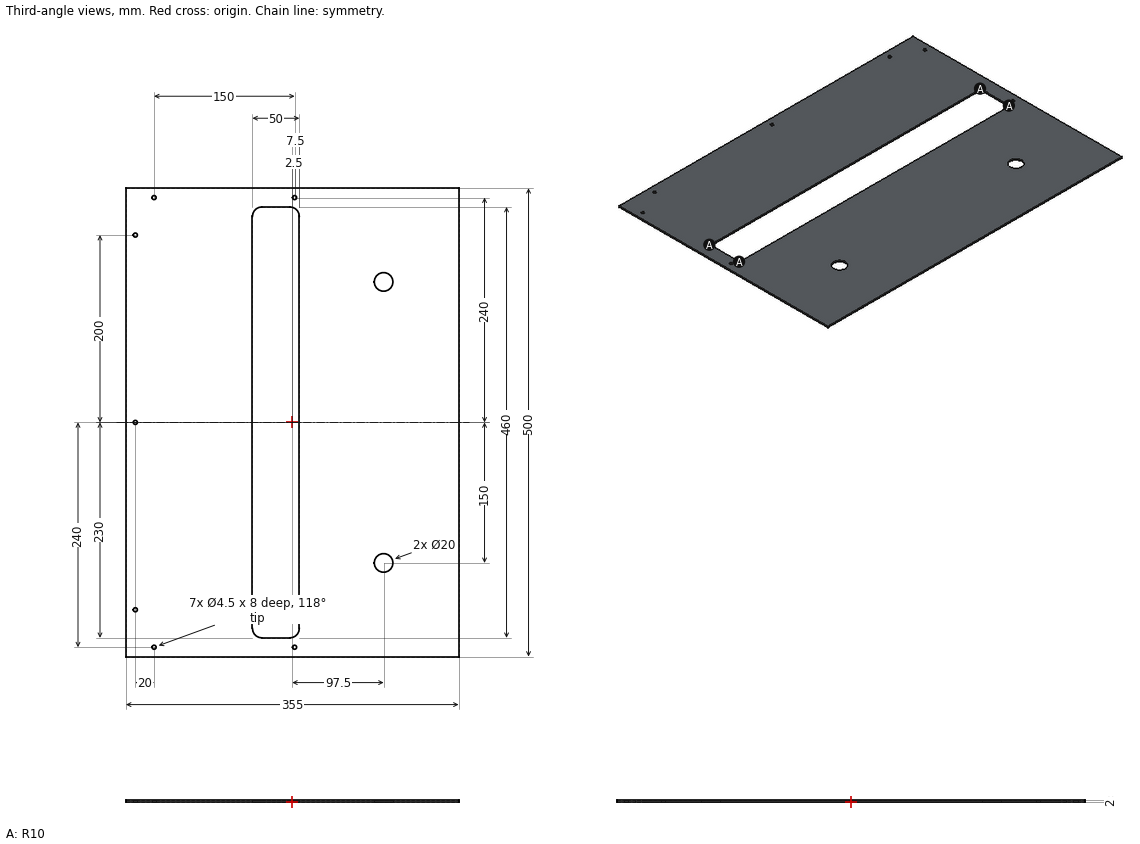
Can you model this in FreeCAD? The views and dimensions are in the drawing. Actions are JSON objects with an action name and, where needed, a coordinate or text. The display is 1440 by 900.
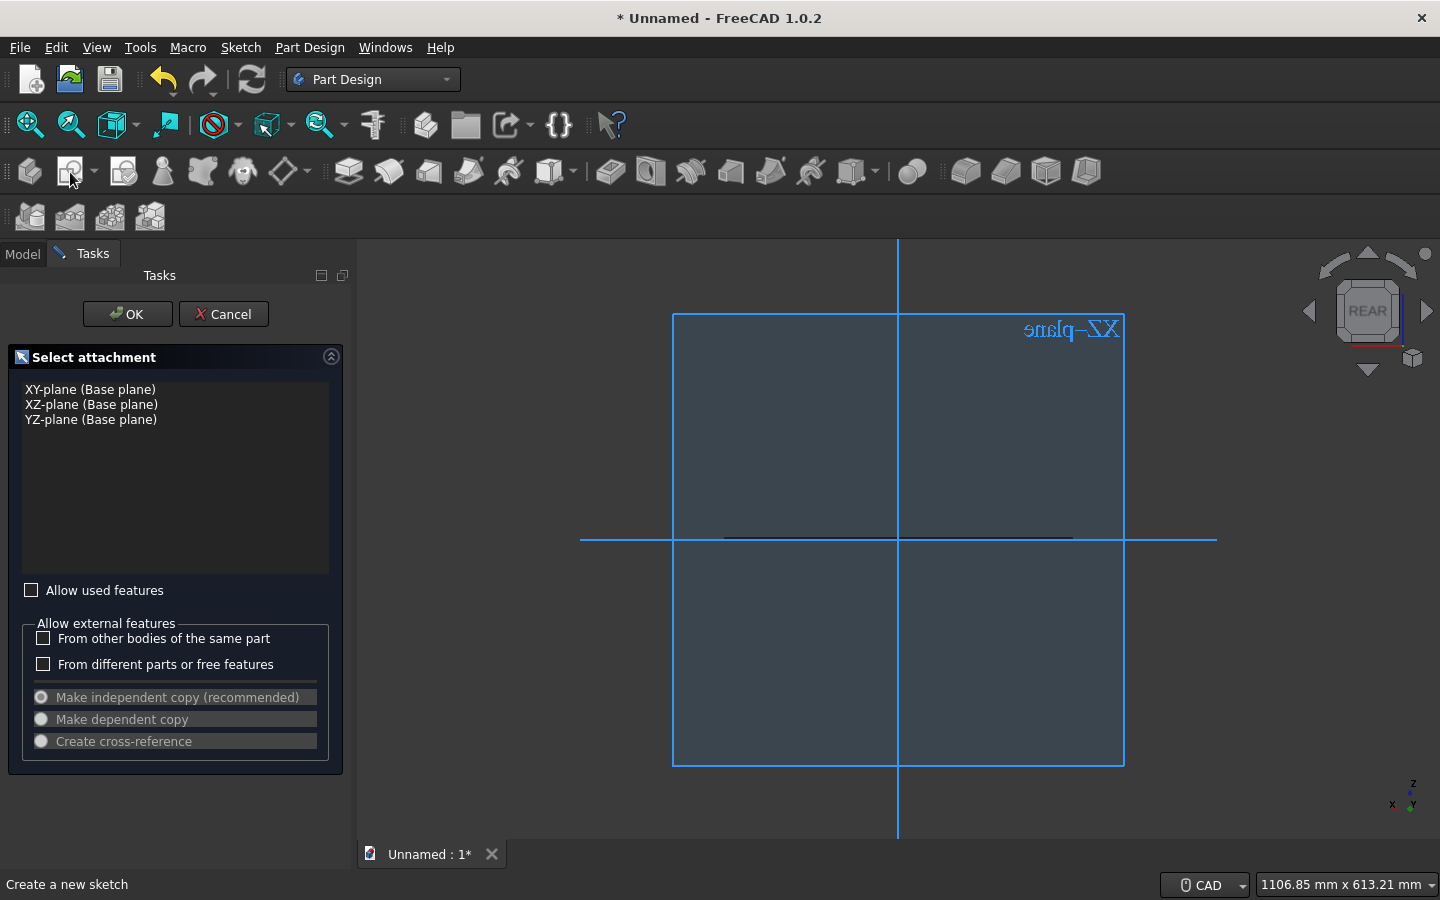
{"action": "left_click", "coordinate": [82, 390]}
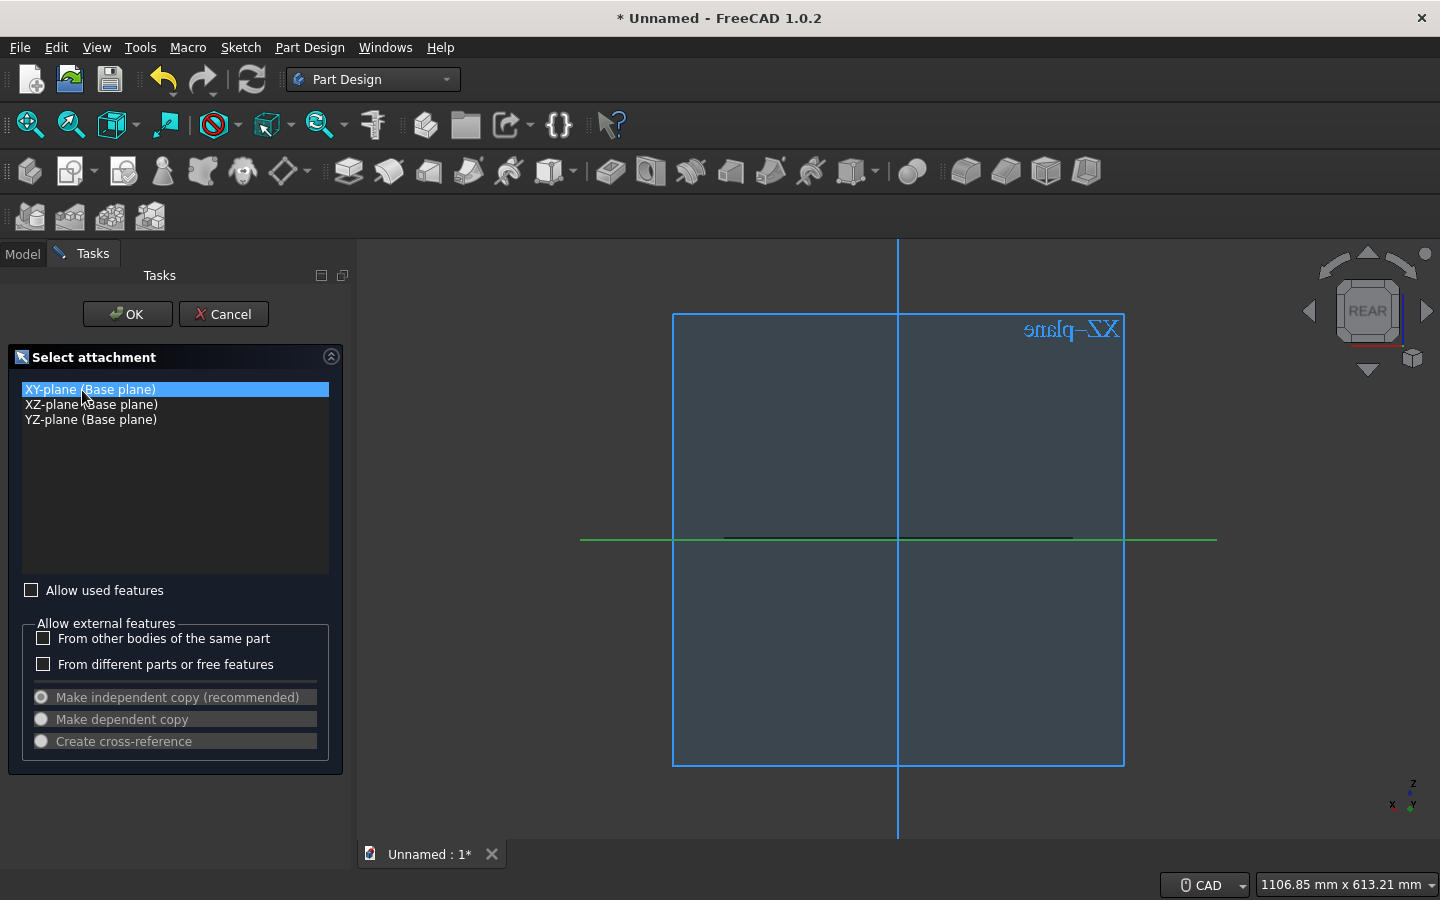
{"action": "left_click", "coordinate": [128, 314]}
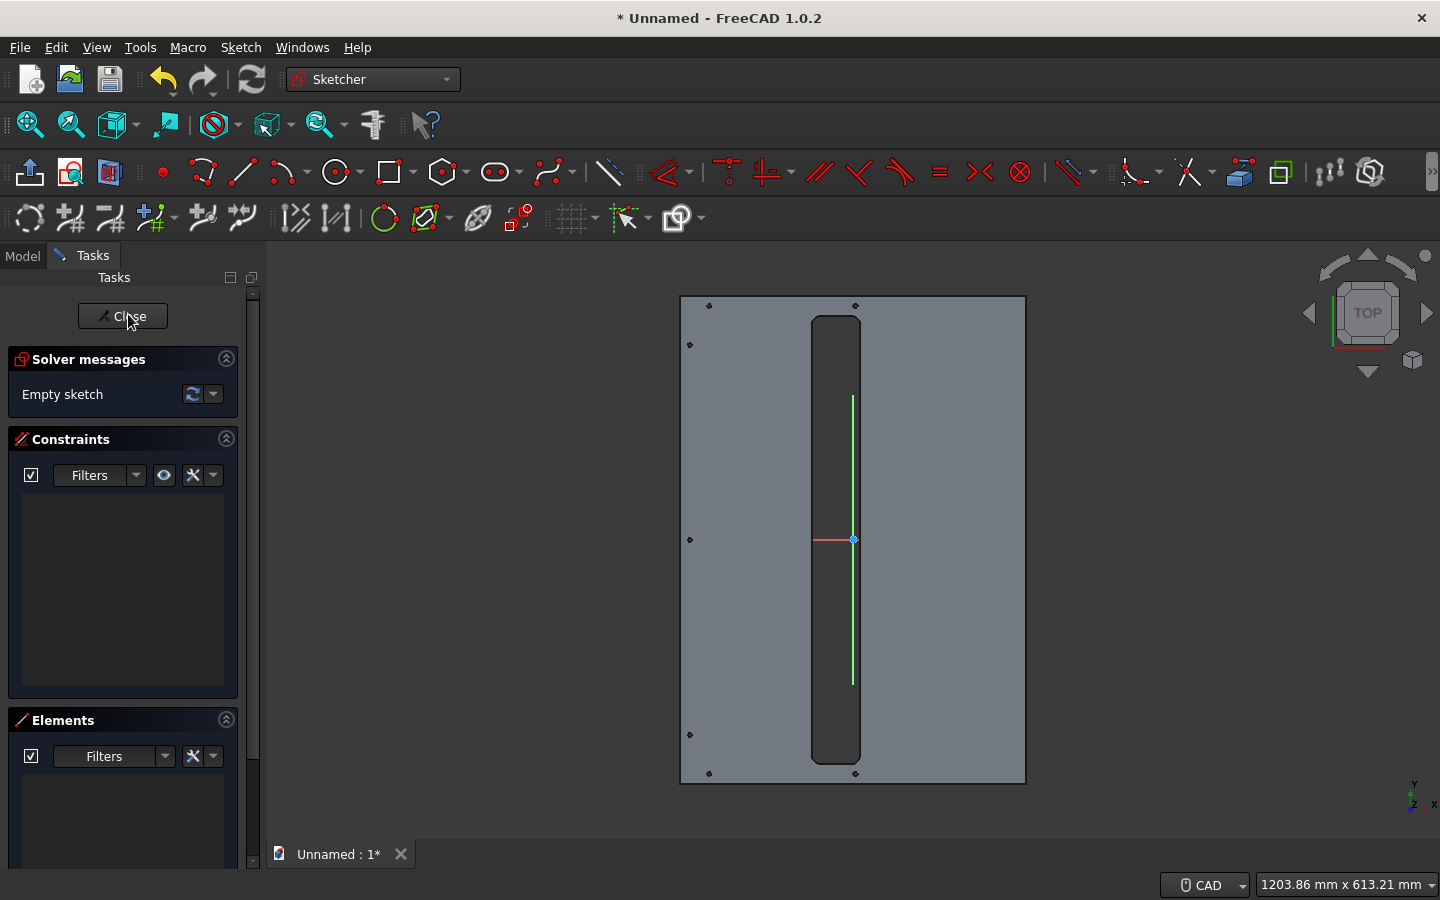
{"action": "left_click", "coordinate": [110, 172]}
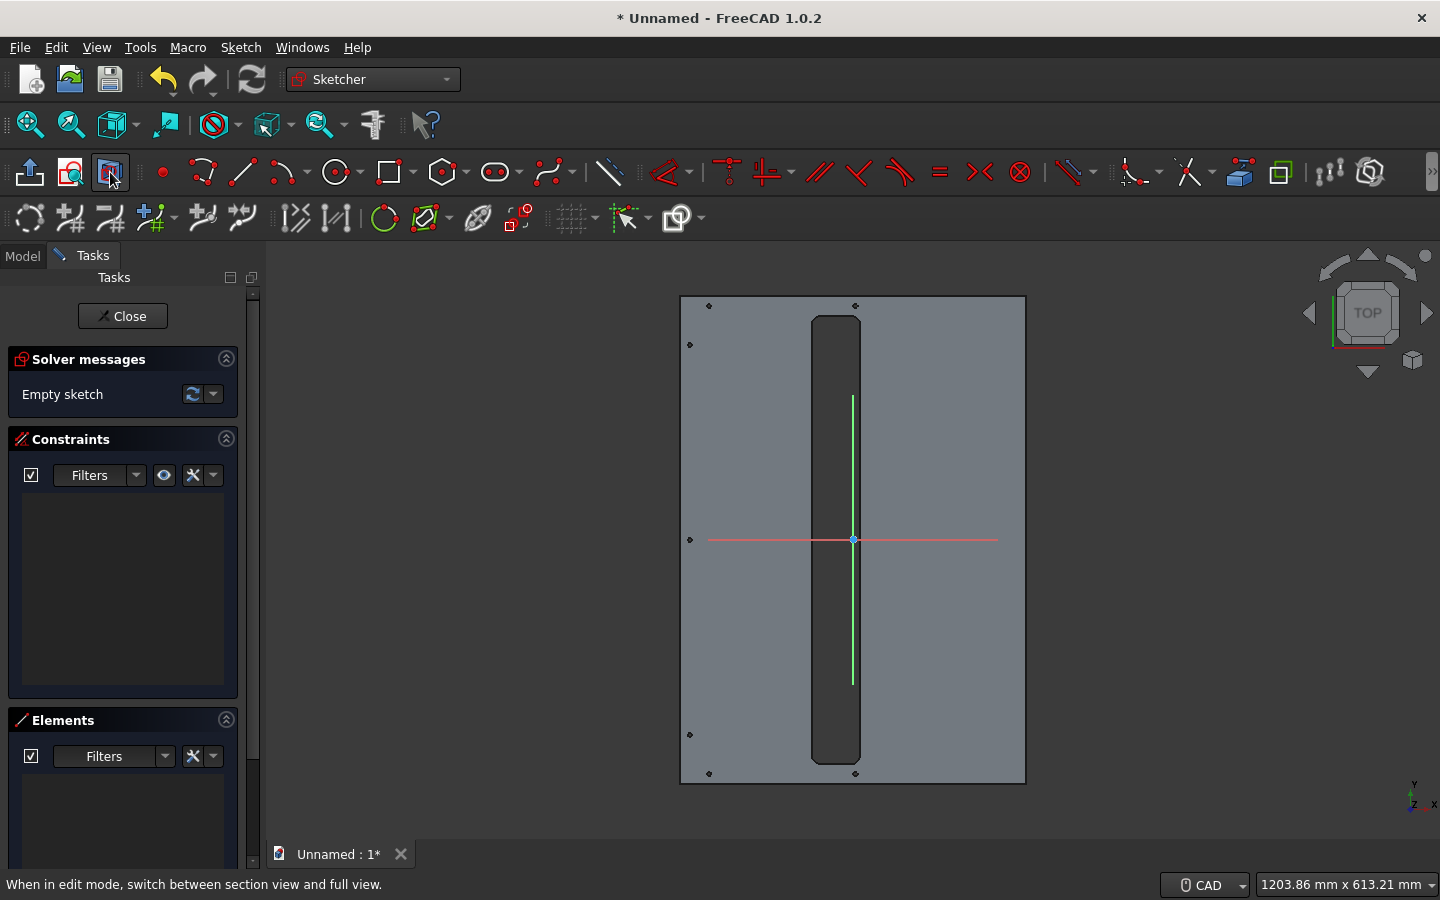
{"action": "left_click", "coordinate": [336, 172]}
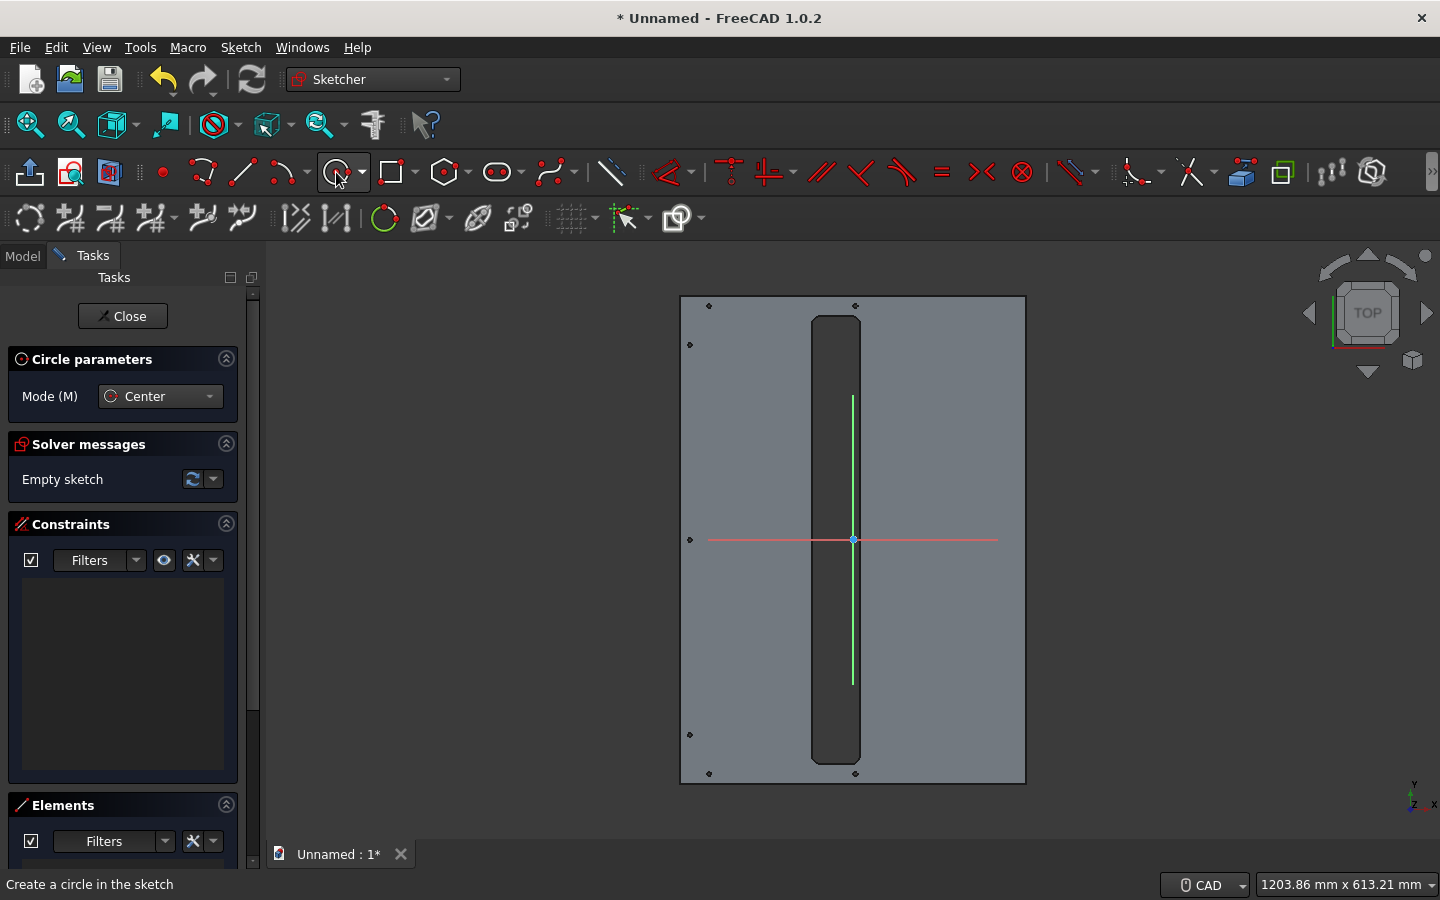
{"action": "scroll", "coordinate": [948, 686], "scroll_direction": "up", "scroll_amount": 5}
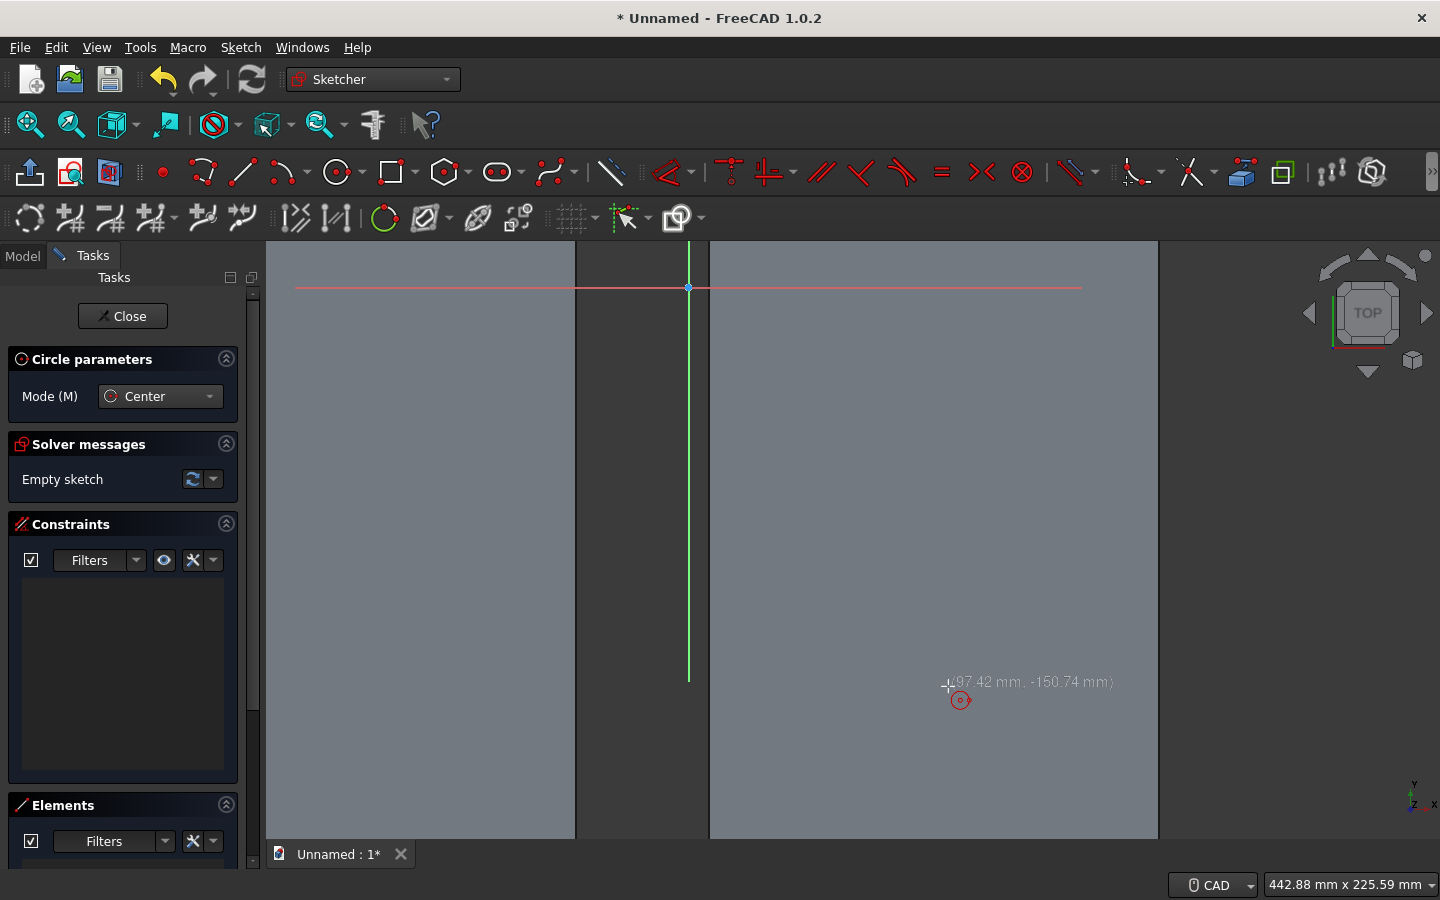
{"action": "left_click", "coordinate": [947, 685]}
{"action": "mouse_move", "coordinate": [966, 667]}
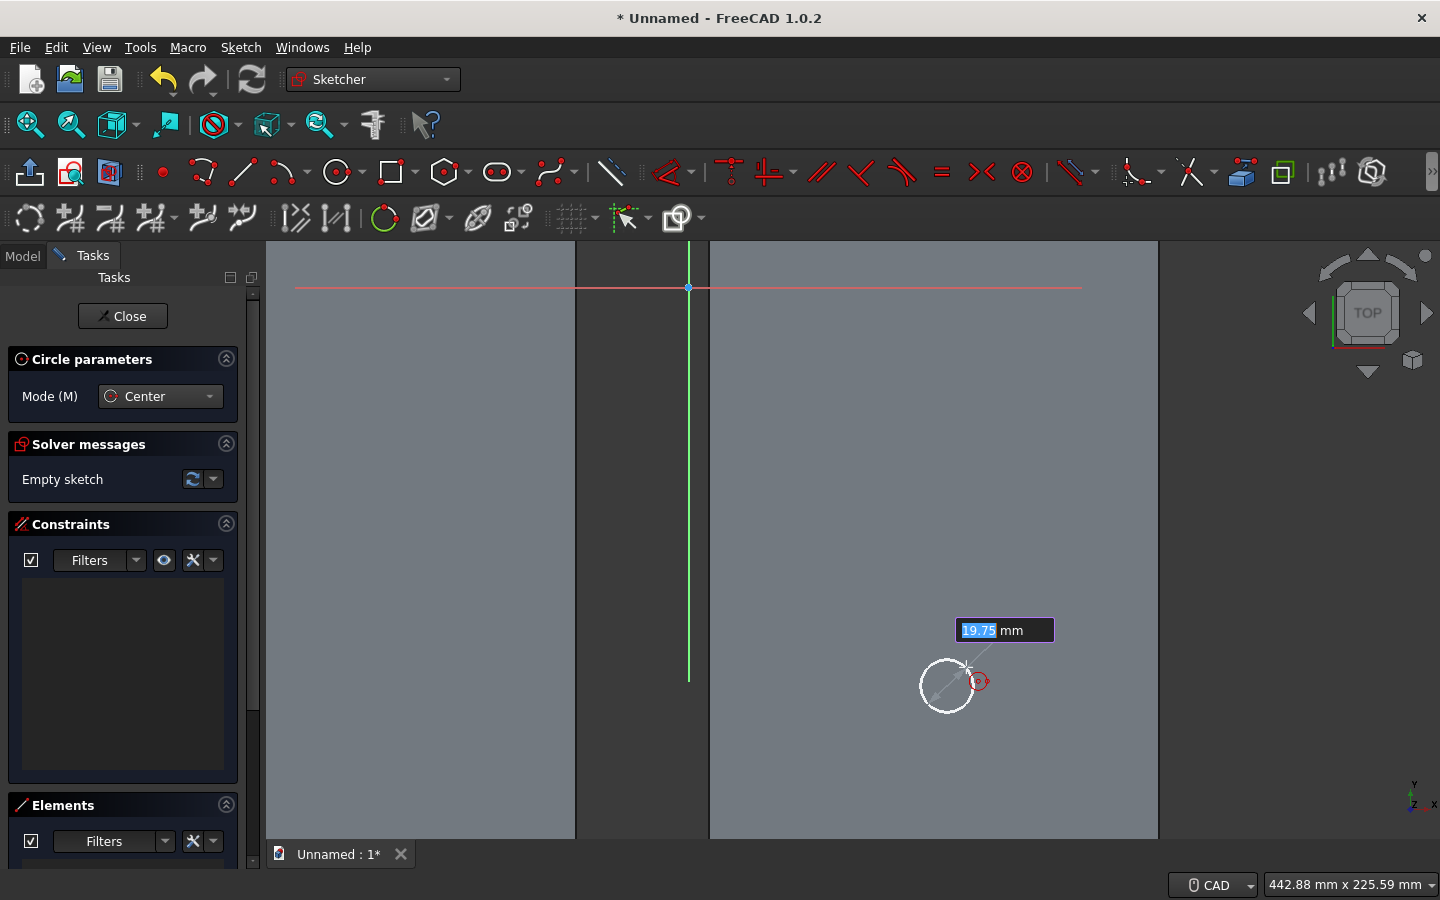
{"action": "type", "text": "20"}
{"action": "key", "text": "Return"}